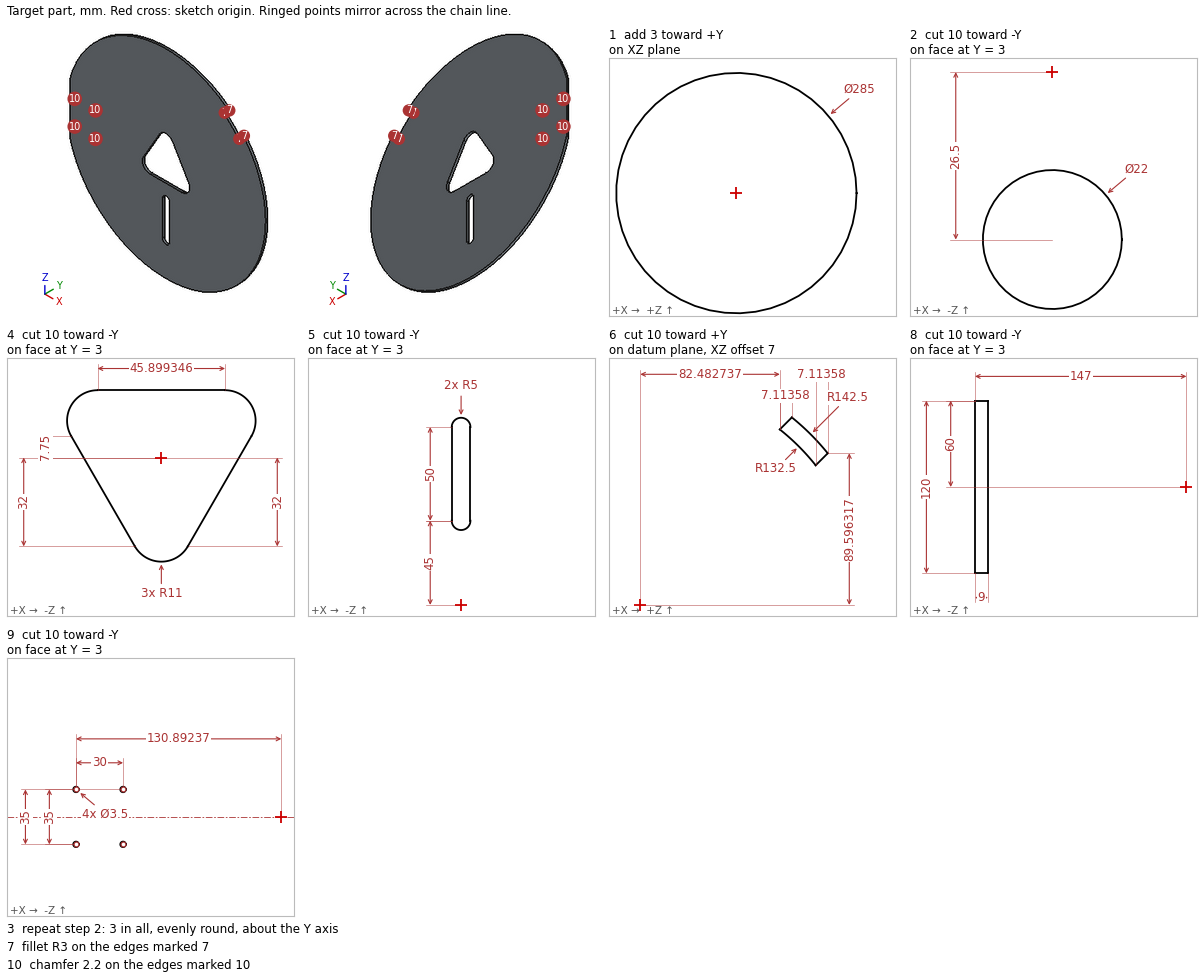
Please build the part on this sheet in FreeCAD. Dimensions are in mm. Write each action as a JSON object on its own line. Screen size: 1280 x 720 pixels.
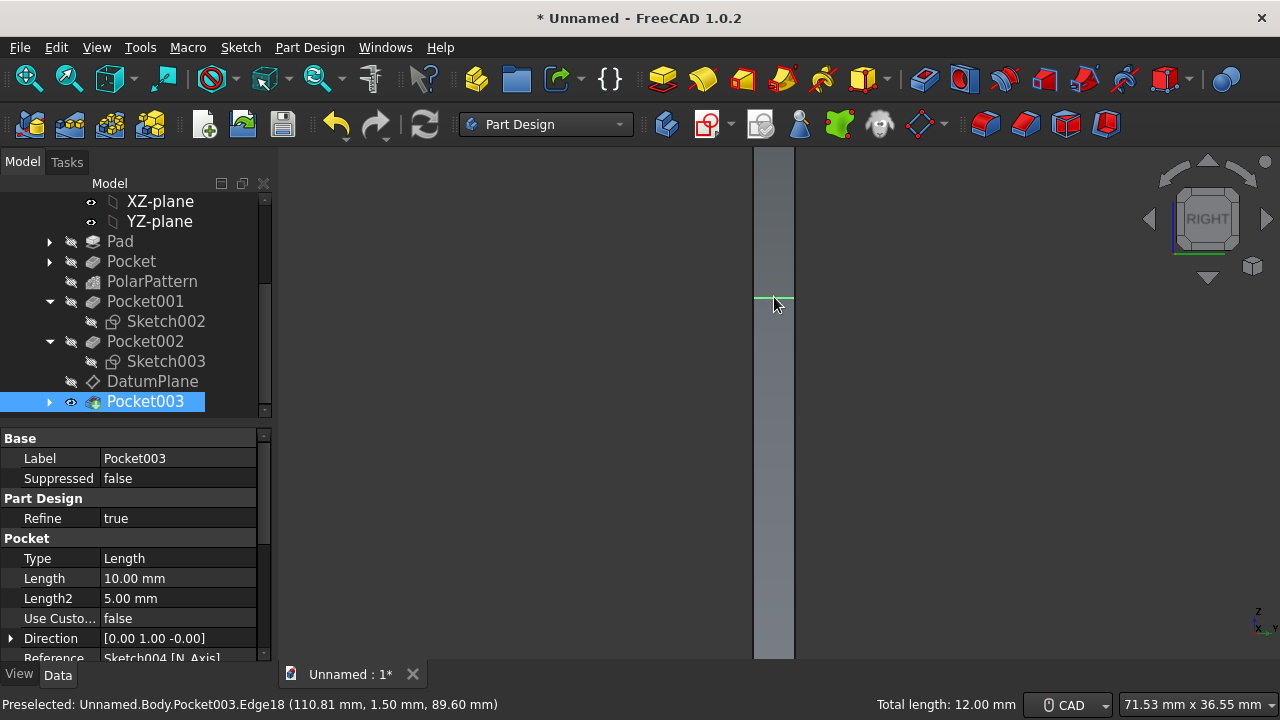
{"action": "left_click", "coordinate": [986, 124]}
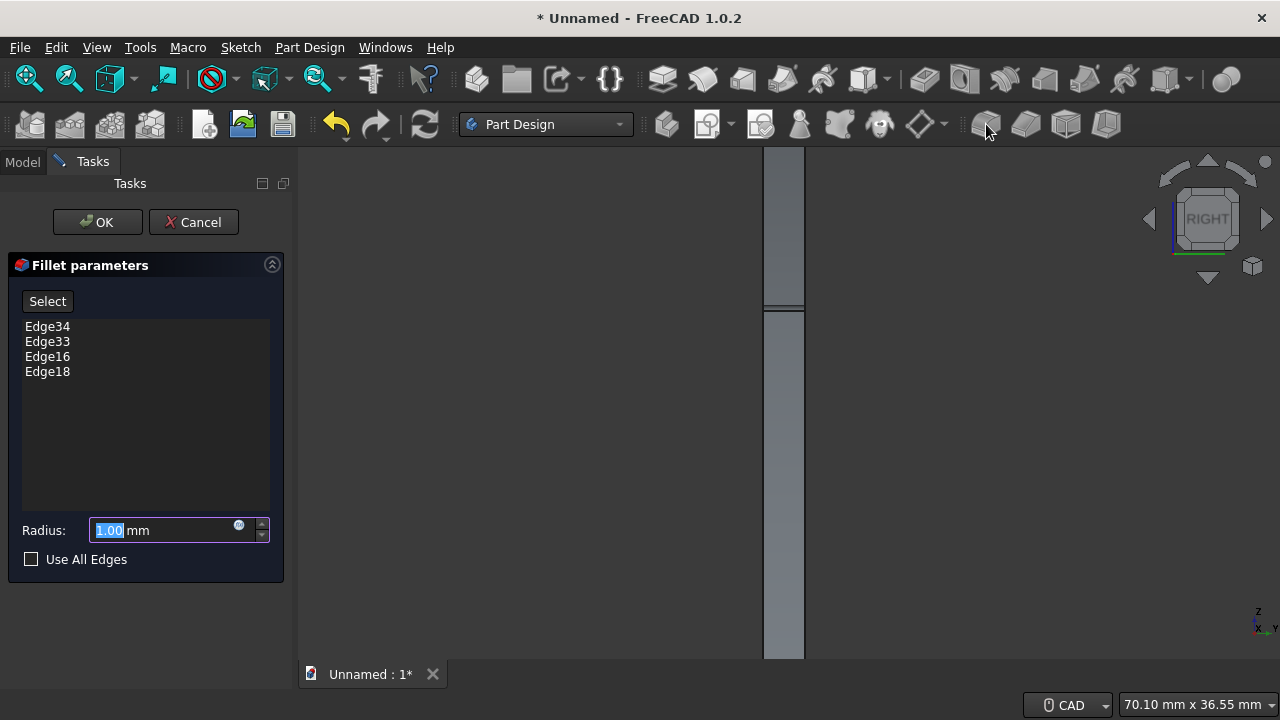
{"action": "type", "text": "3"}
{"action": "key", "text": "Tab"}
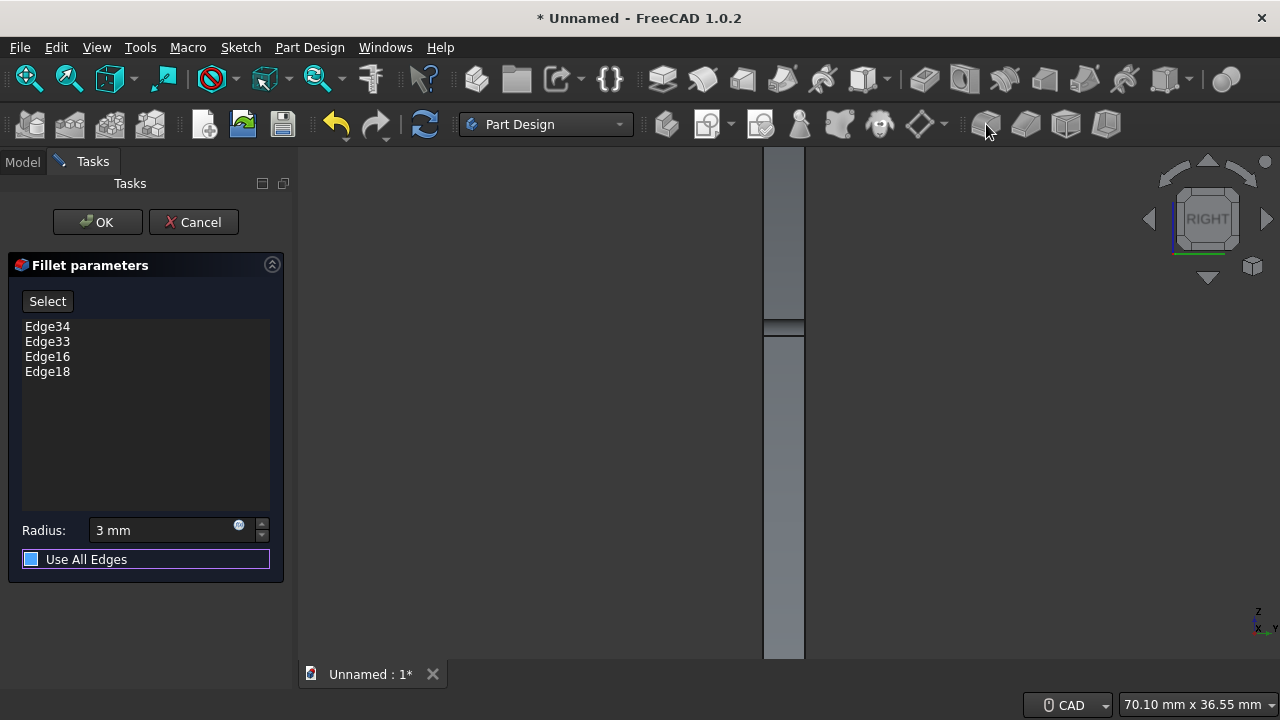
{"action": "left_click", "coordinate": [98, 222]}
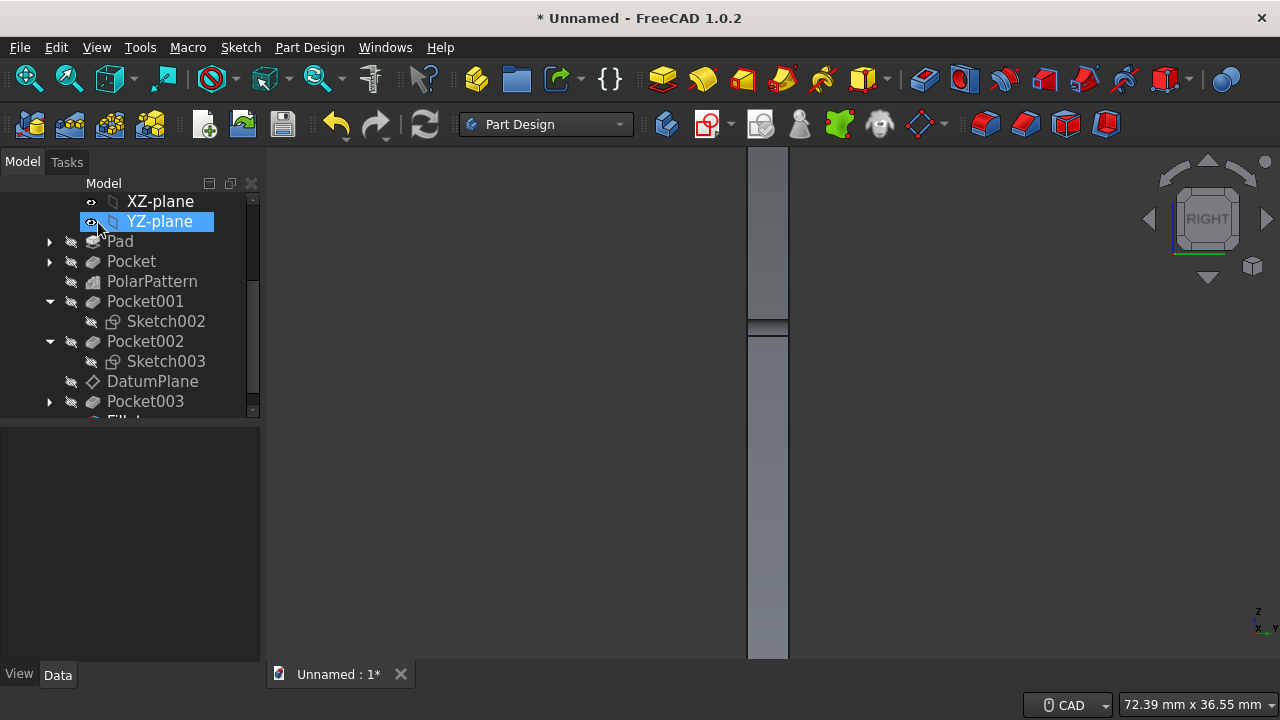
{"action": "left_click", "coordinate": [30, 80]}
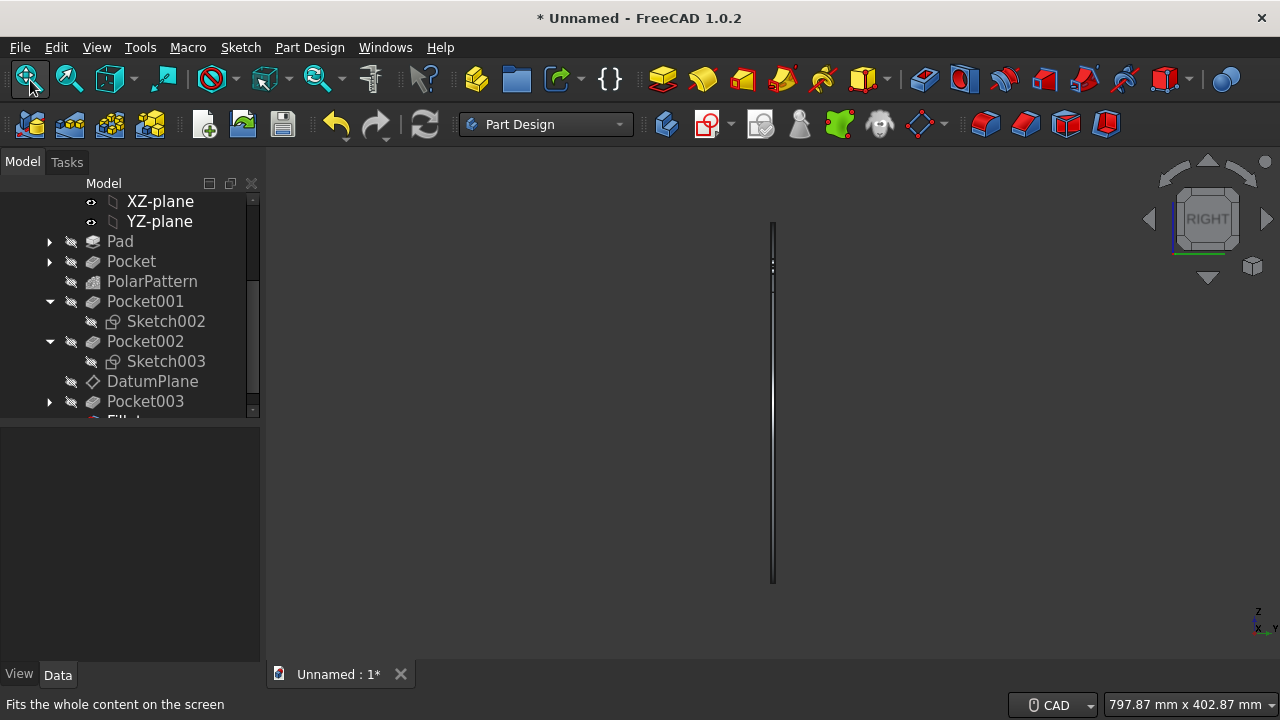
{"action": "key", "text": "4"}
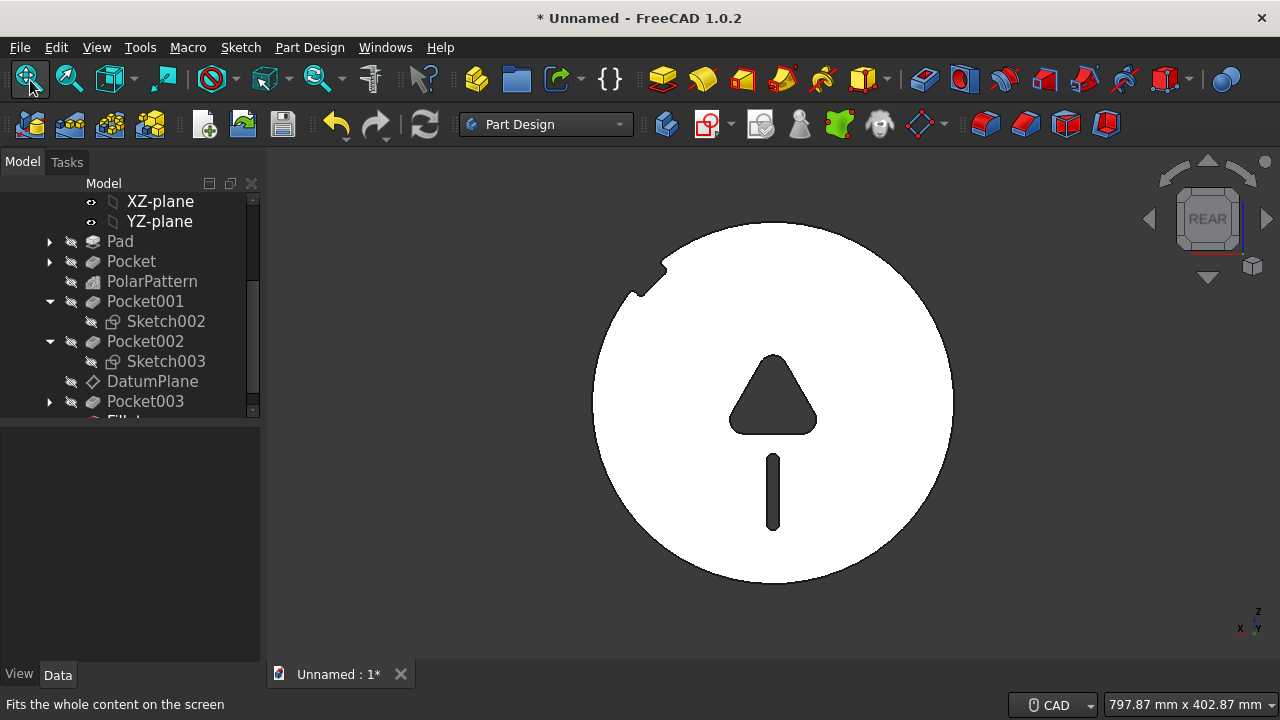
{"action": "left_click", "coordinate": [670, 454]}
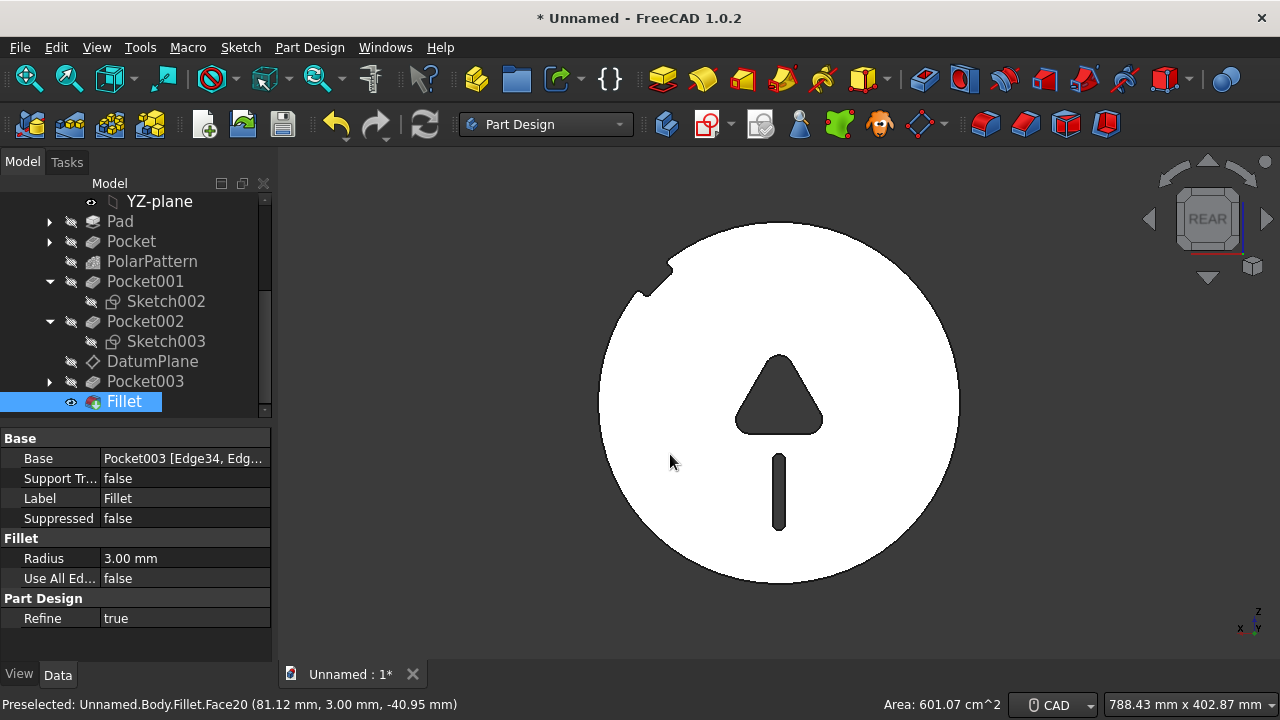
{"action": "left_click", "coordinate": [708, 124]}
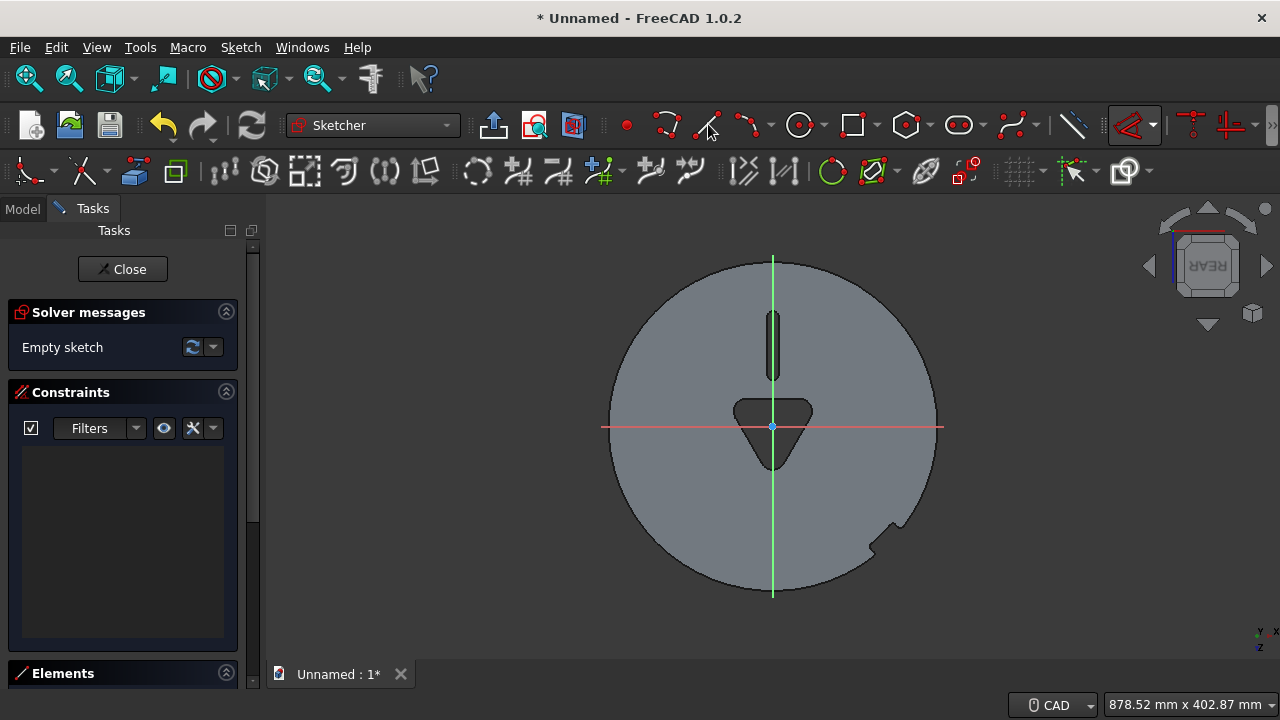
{"action": "scroll", "coordinate": [675, 427], "scroll_direction": "up", "scroll_amount": 4}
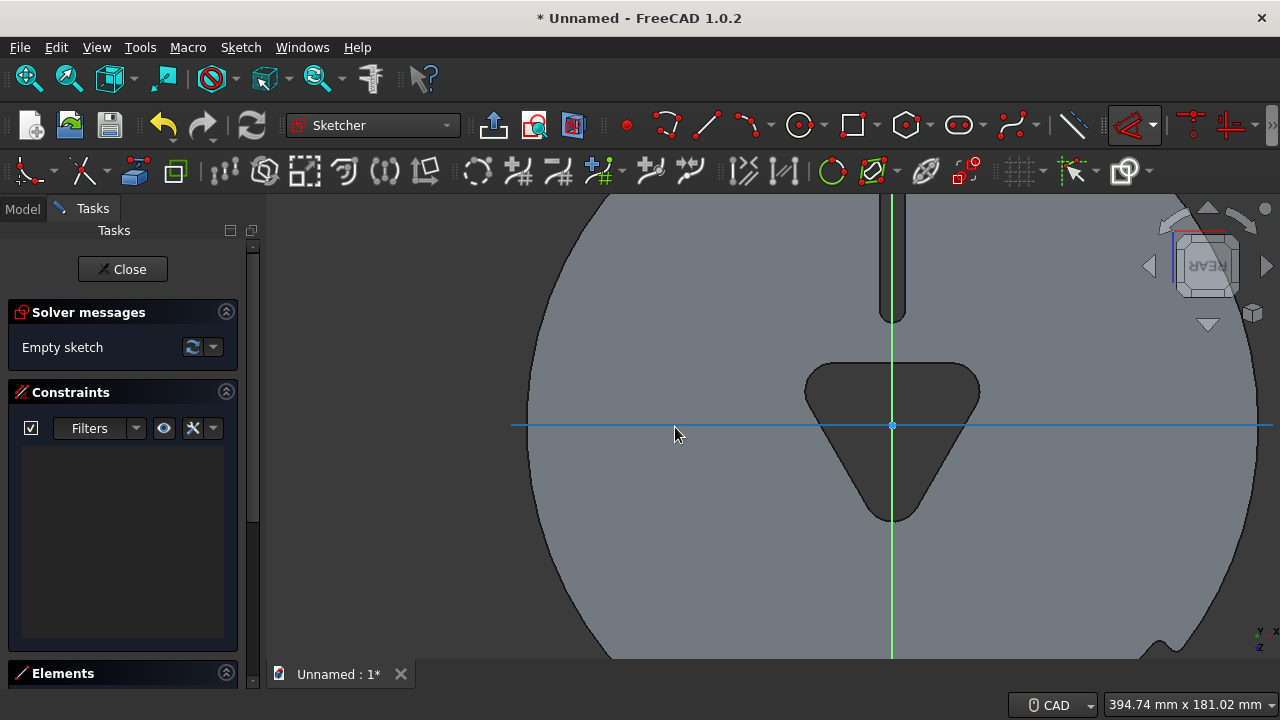
{"action": "left_click", "coordinate": [854, 126]}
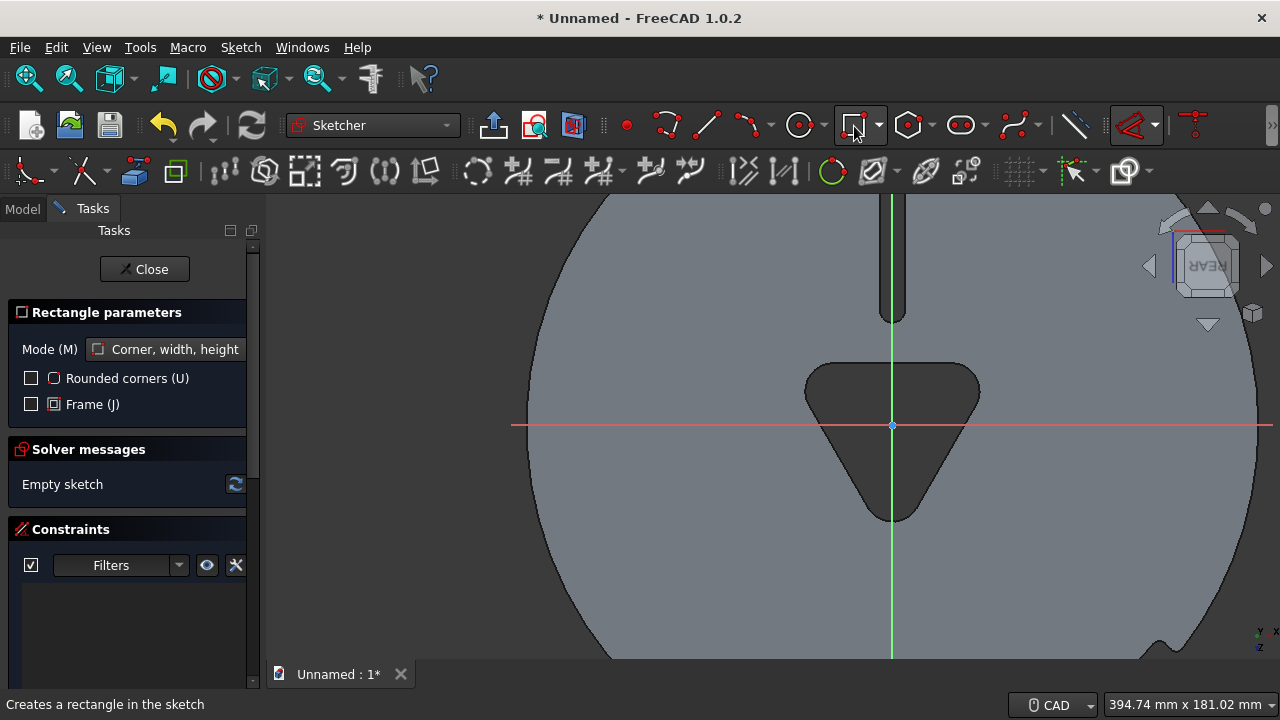
{"action": "left_click", "coordinate": [515, 271]}
{"action": "left_click", "coordinate": [538, 579]}
{"action": "key", "text": "Escape"}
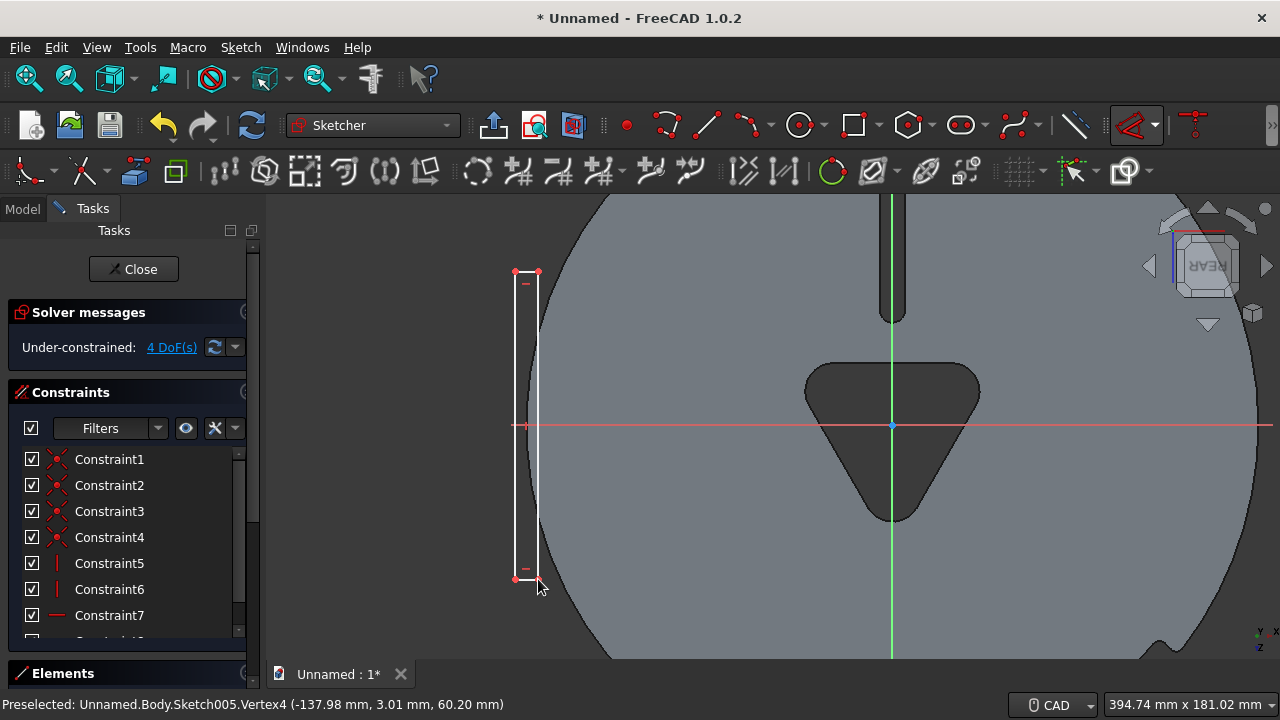
{"action": "scroll", "coordinate": [524, 580], "scroll_direction": "up", "scroll_amount": 3}